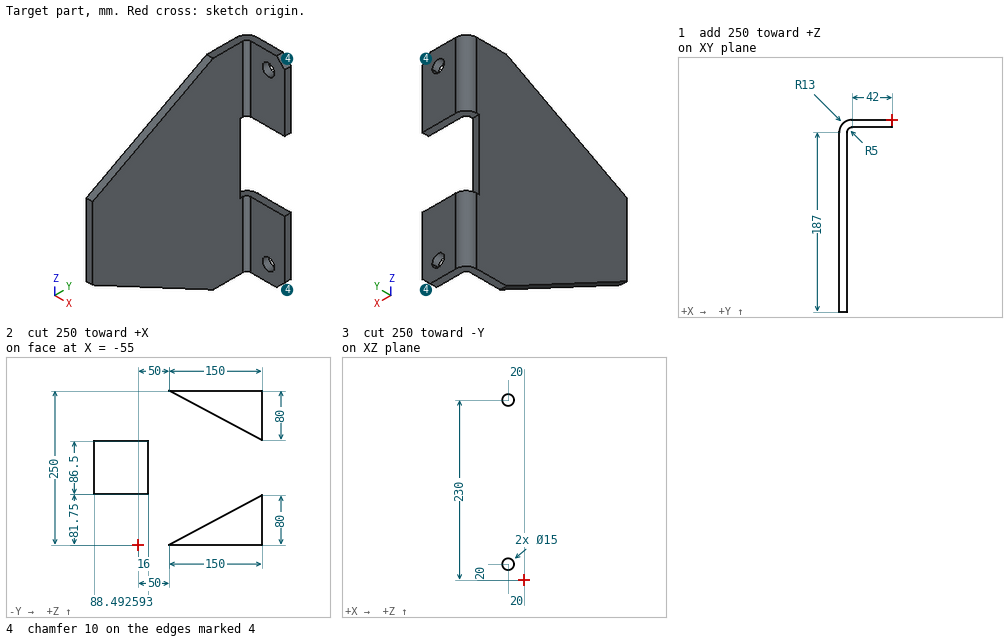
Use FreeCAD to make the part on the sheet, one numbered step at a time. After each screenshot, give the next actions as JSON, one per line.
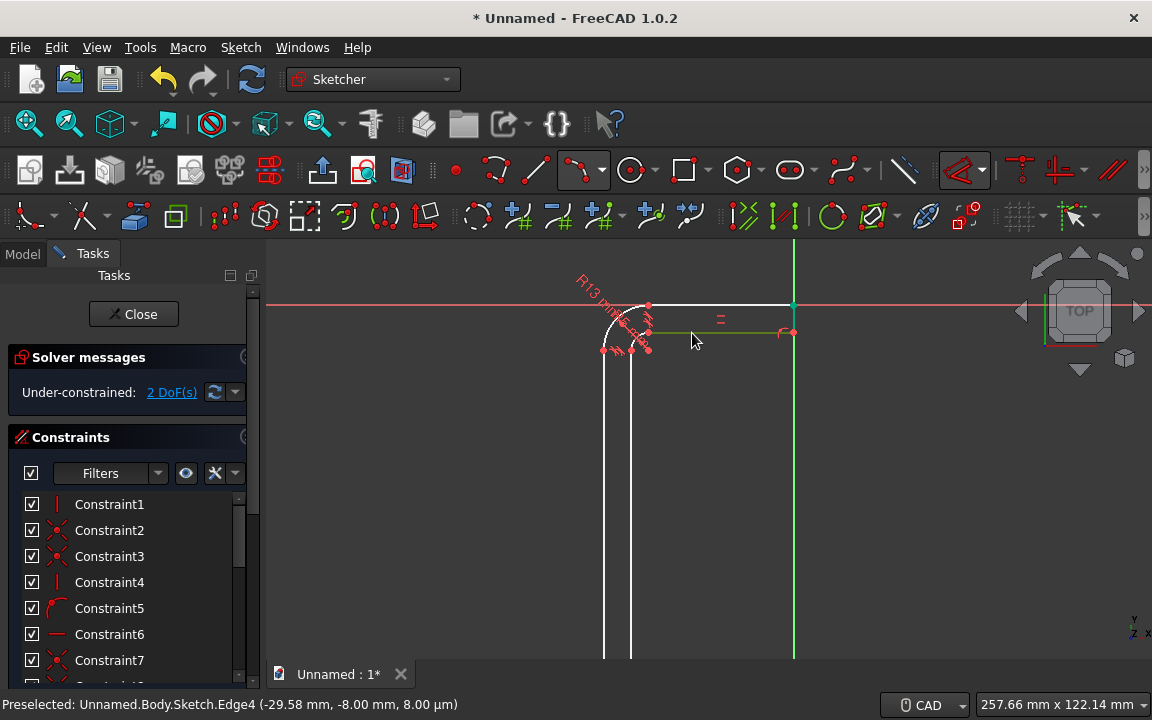
{"action": "key", "text": "l"}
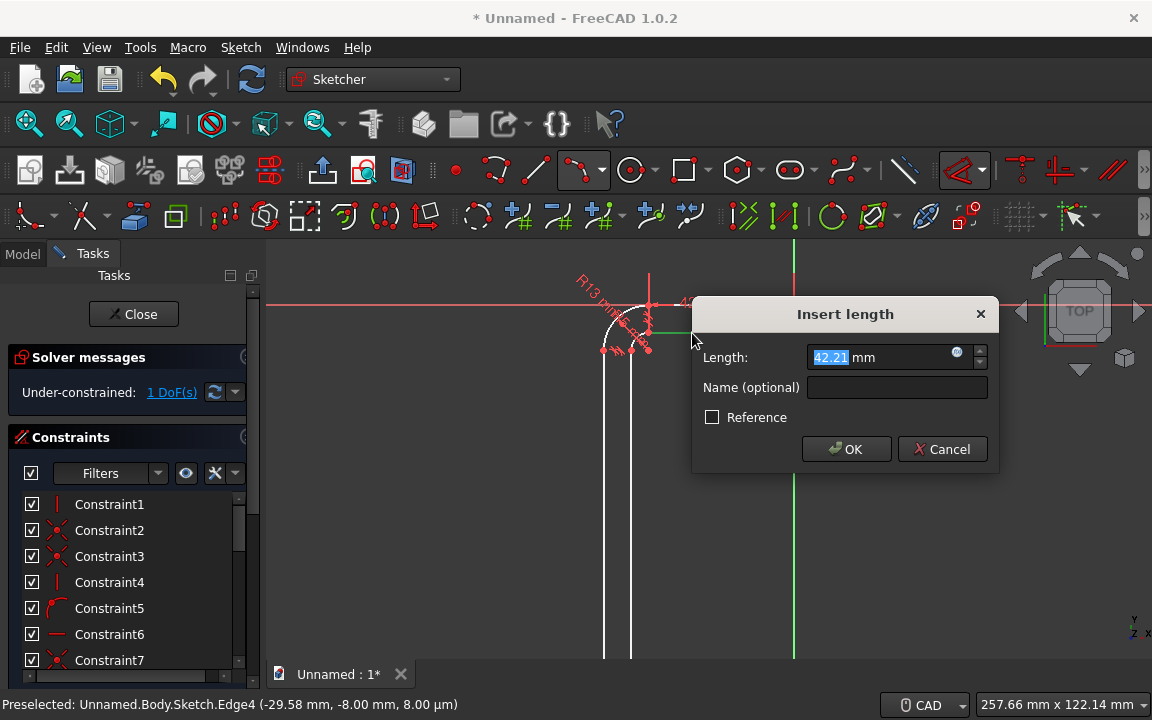
{"action": "type", "text": "42"}
{"action": "key", "text": "Return"}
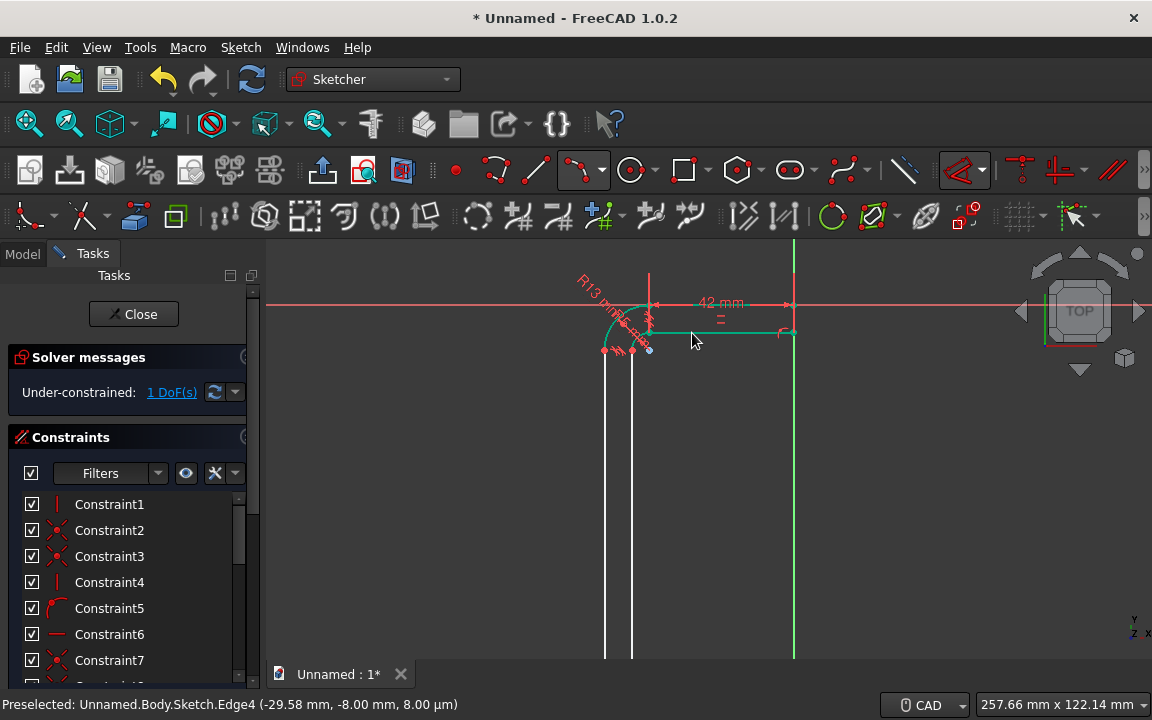
{"action": "left_click", "coordinate": [605, 544]}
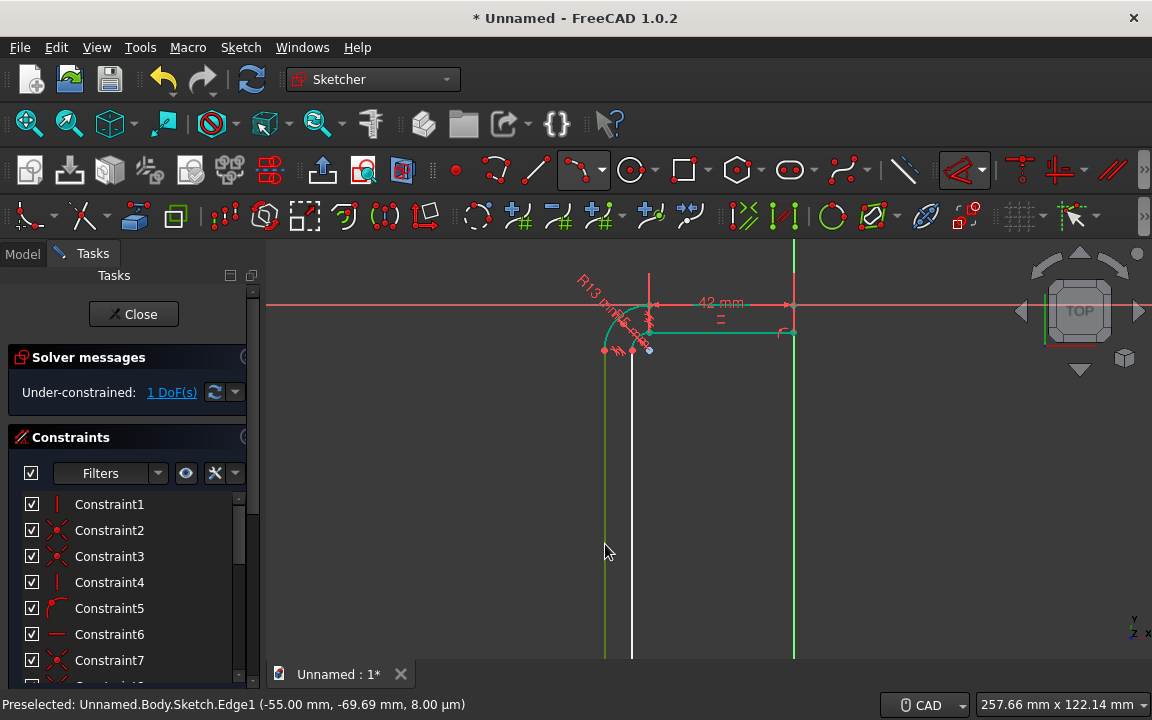
{"action": "left_click", "coordinate": [984, 170]}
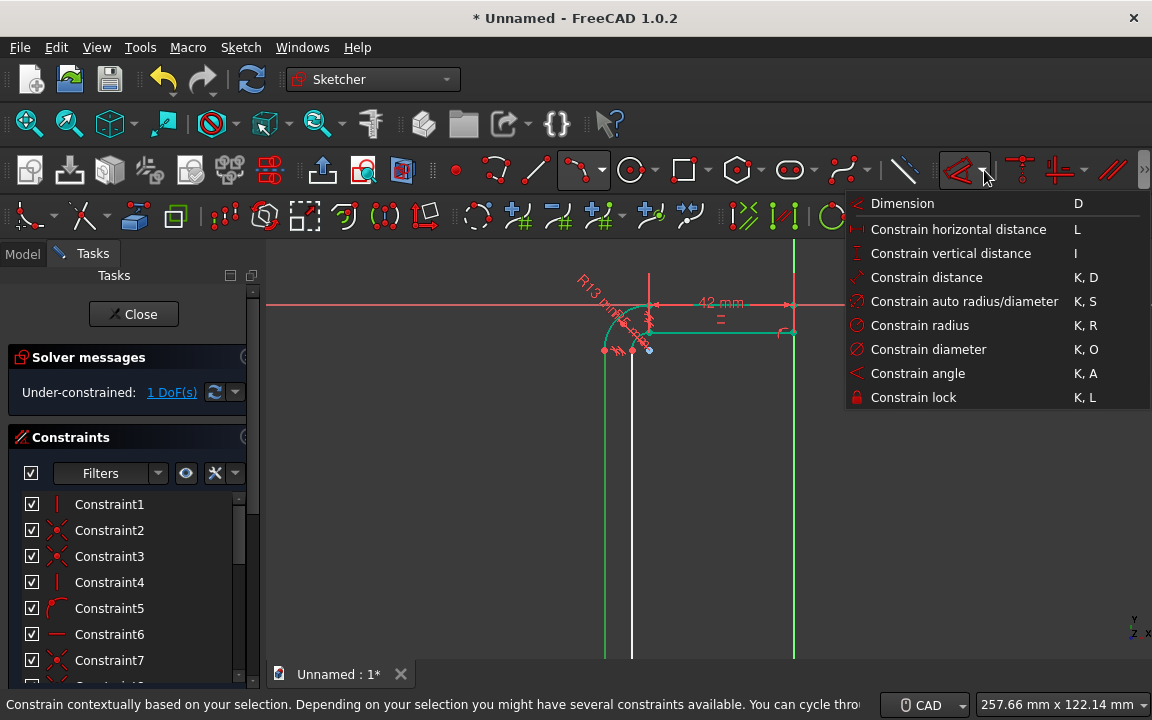
{"action": "left_click", "coordinate": [998, 253]}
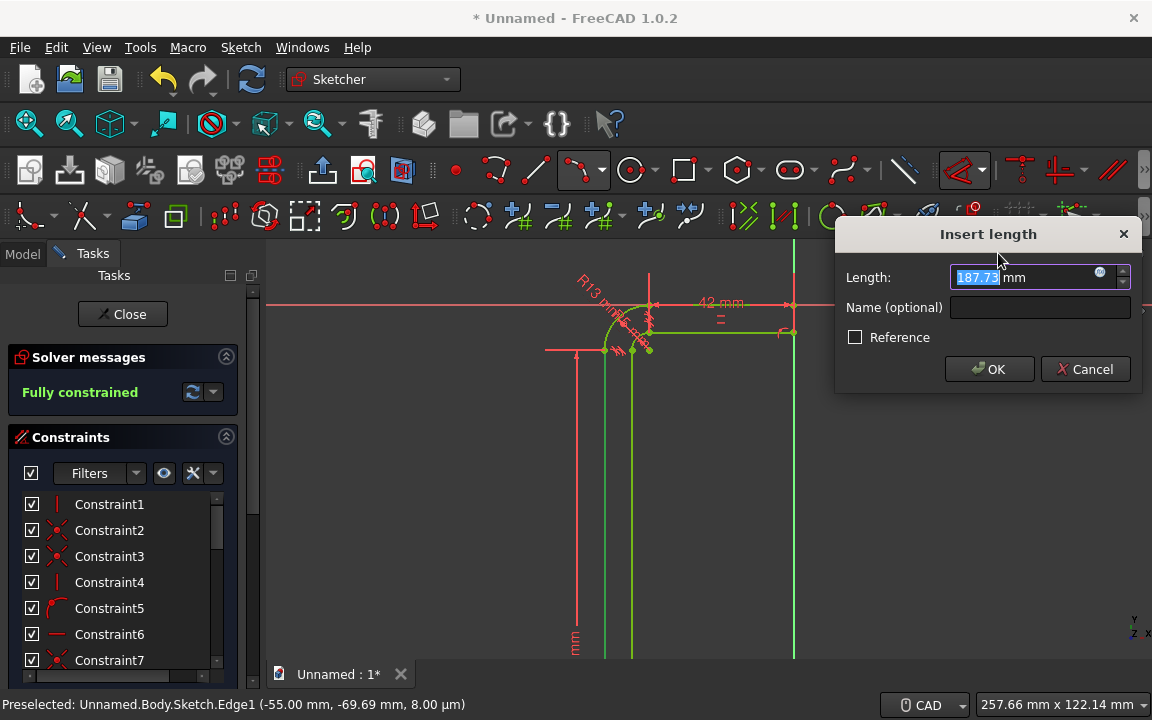
{"action": "type", "text": "187"}
{"action": "key", "text": "Return"}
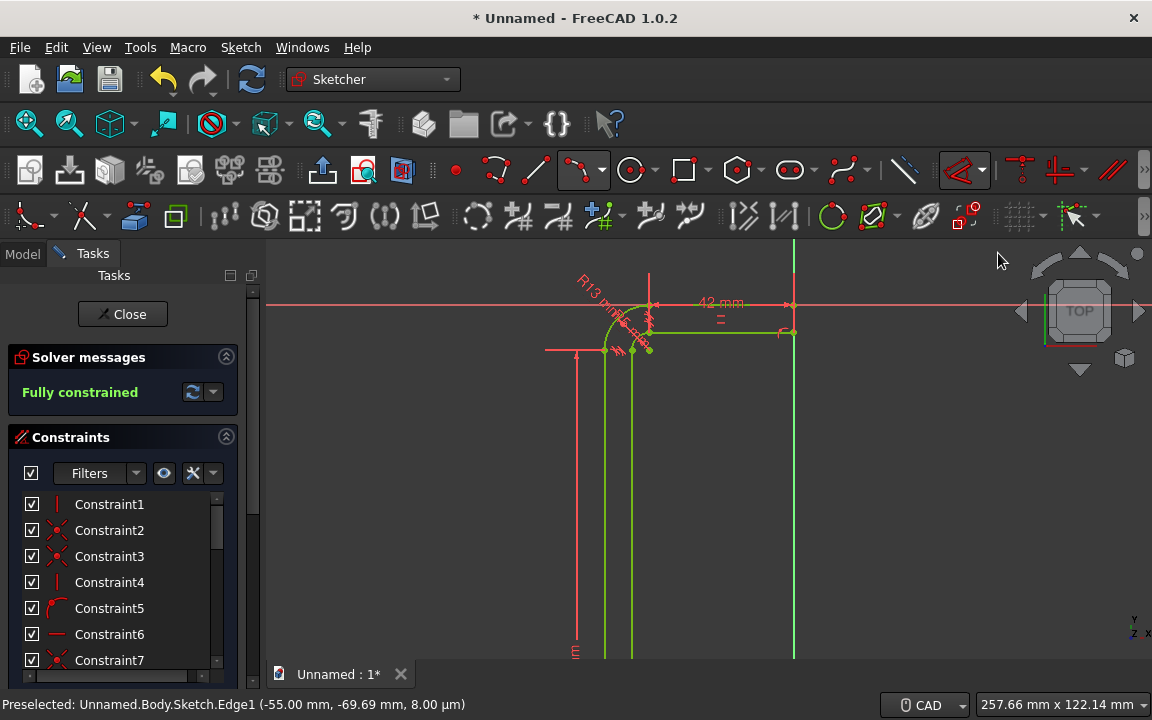
{"action": "left_click", "coordinate": [123, 314]}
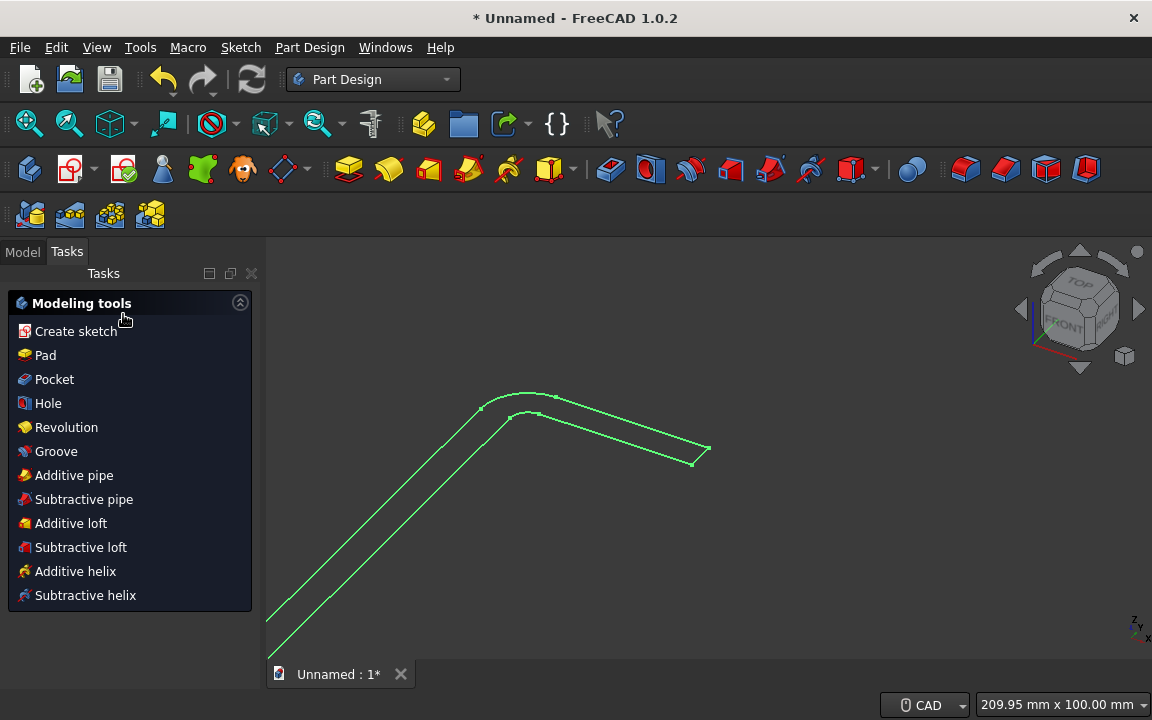
{"action": "left_click", "coordinate": [350, 170]}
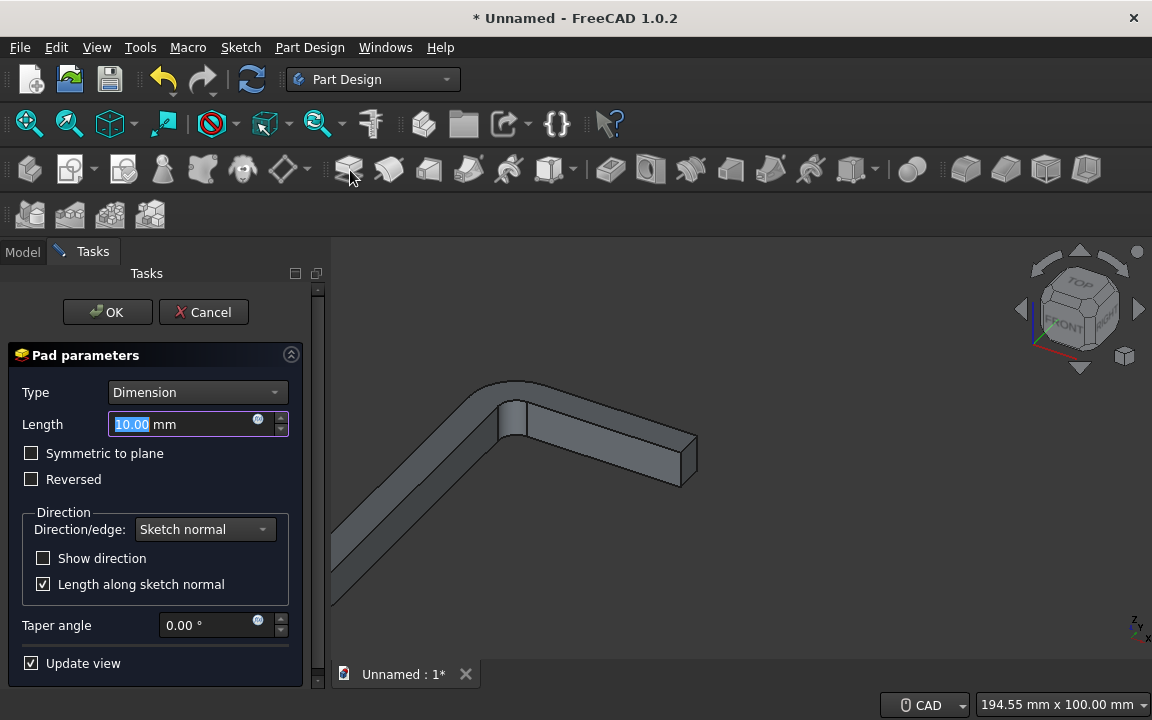
{"action": "type", "text": "250"}
{"action": "key", "text": "Tab"}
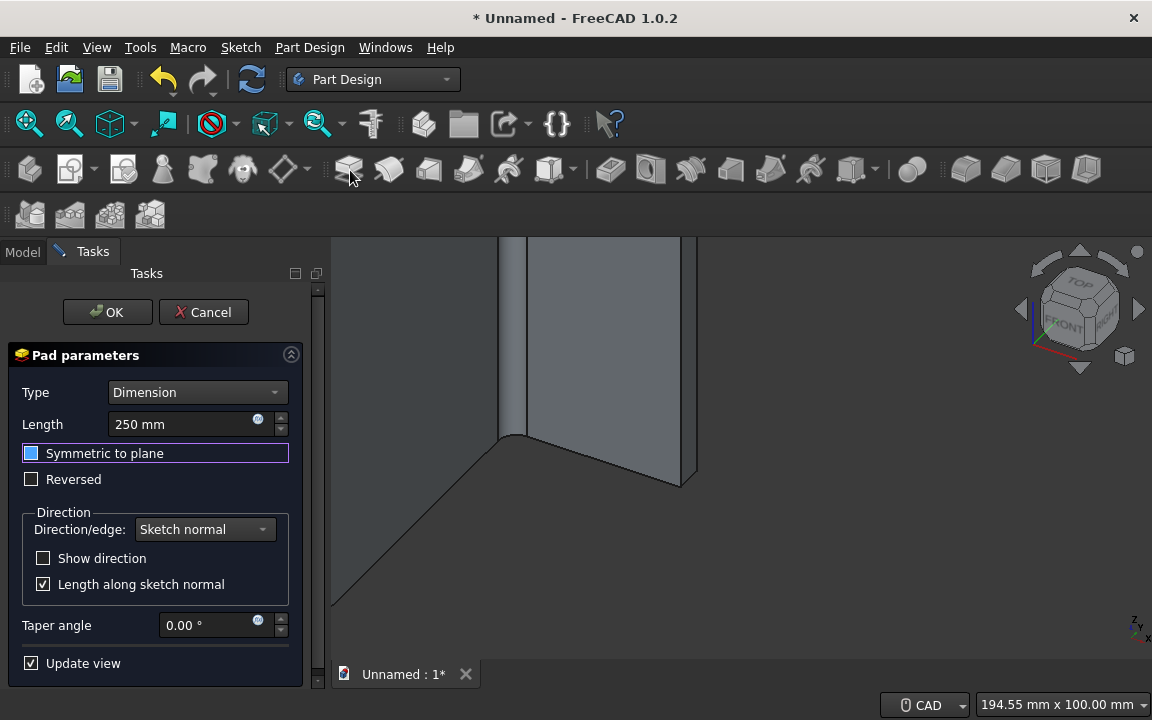
{"action": "left_click", "coordinate": [108, 312]}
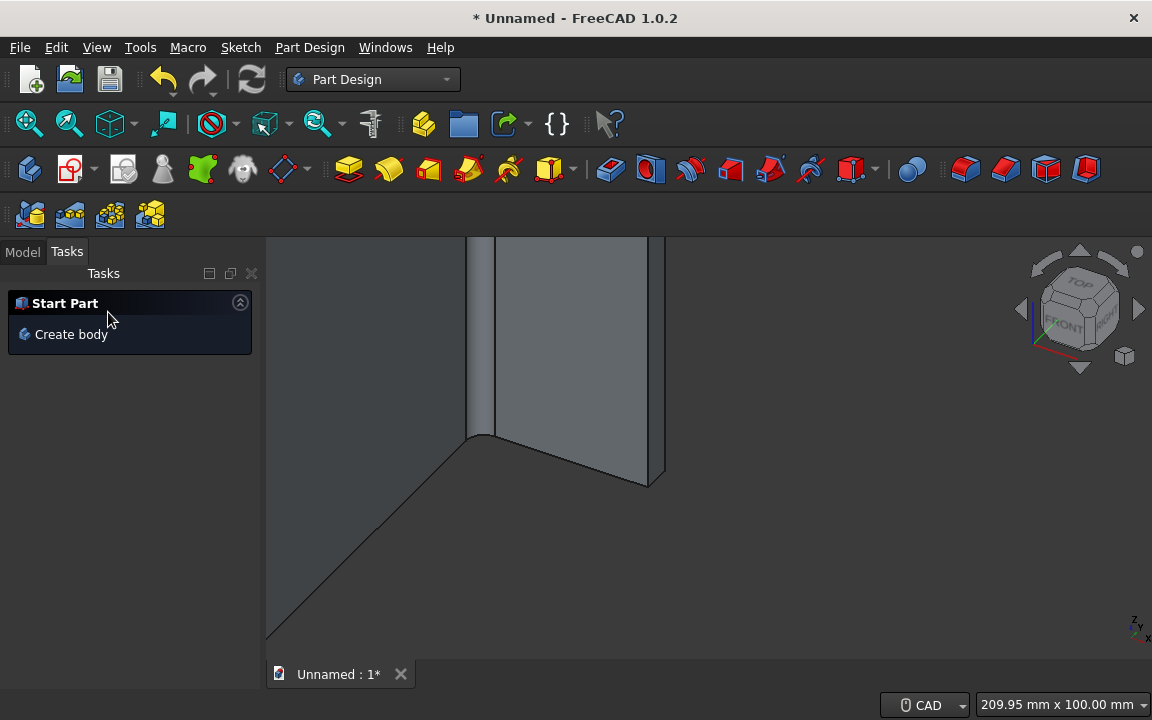
{"action": "key", "text": "v f"}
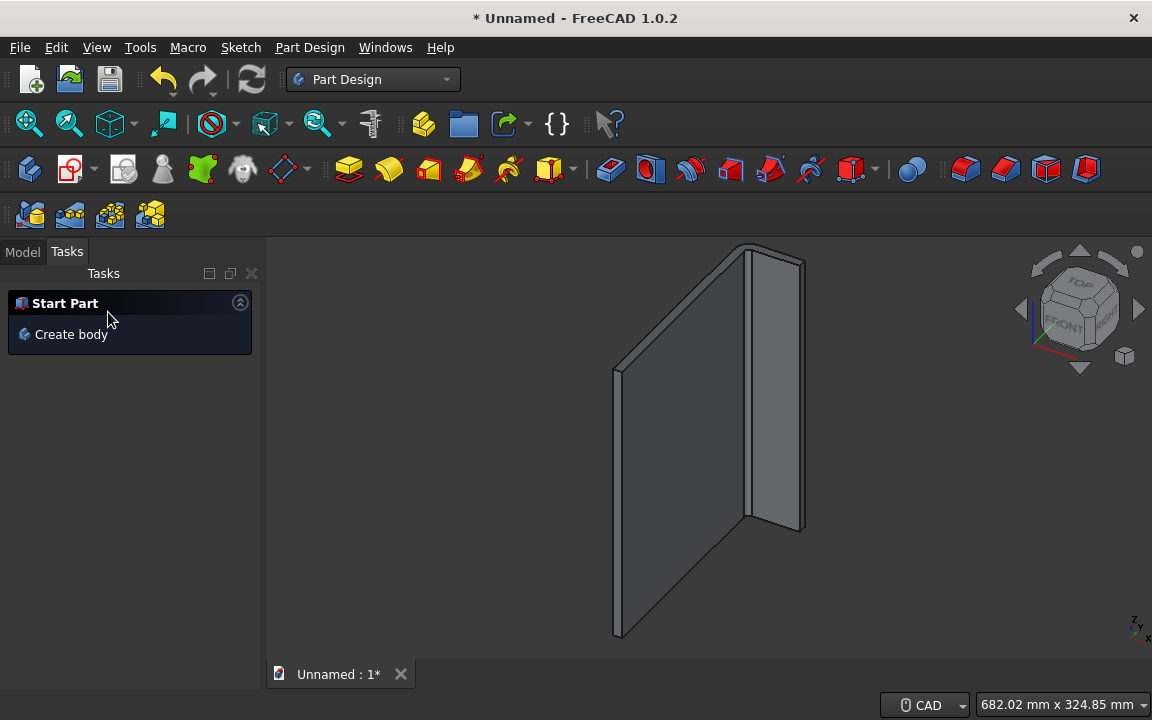
{"action": "key", "text": "6"}